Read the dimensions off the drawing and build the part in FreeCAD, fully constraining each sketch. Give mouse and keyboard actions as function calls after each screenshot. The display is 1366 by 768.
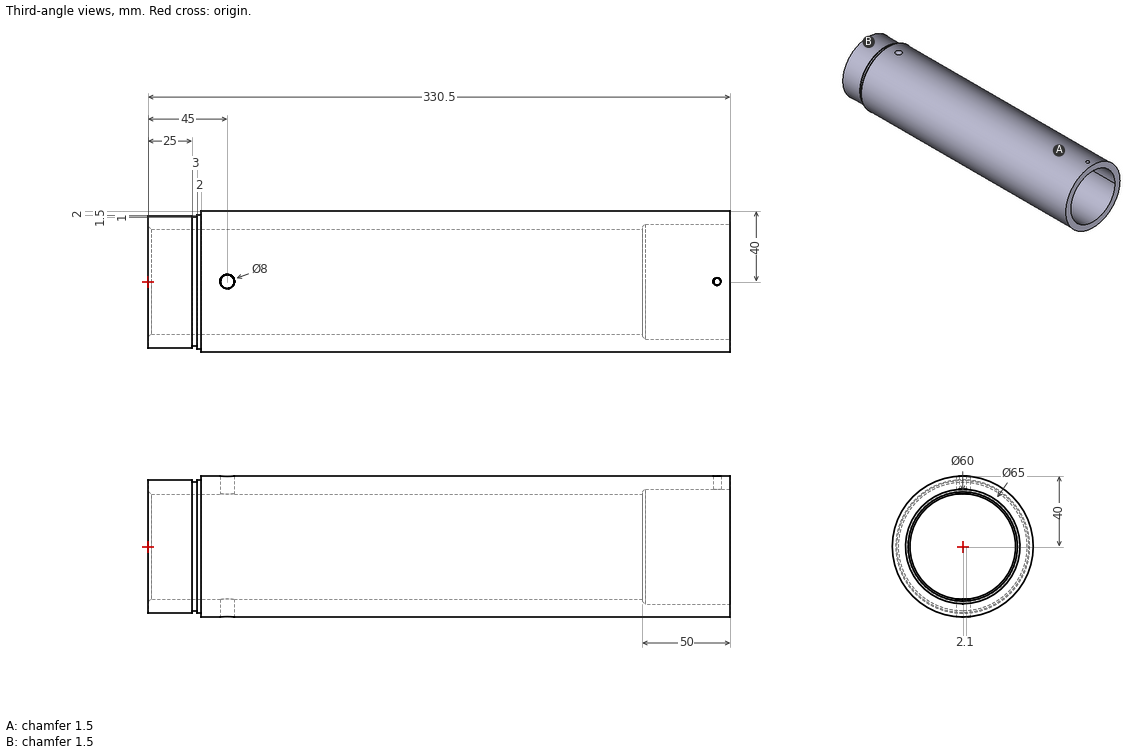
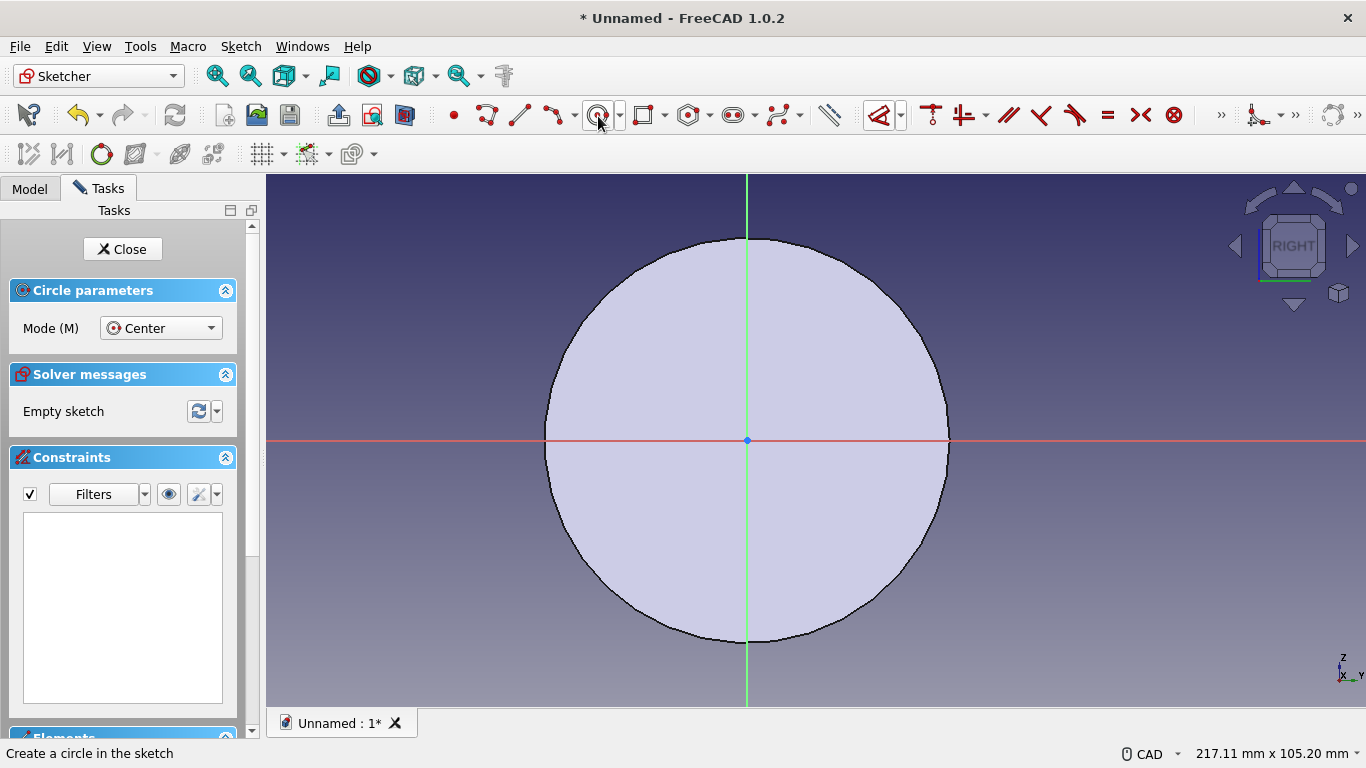
click(747, 440)
move(864, 324)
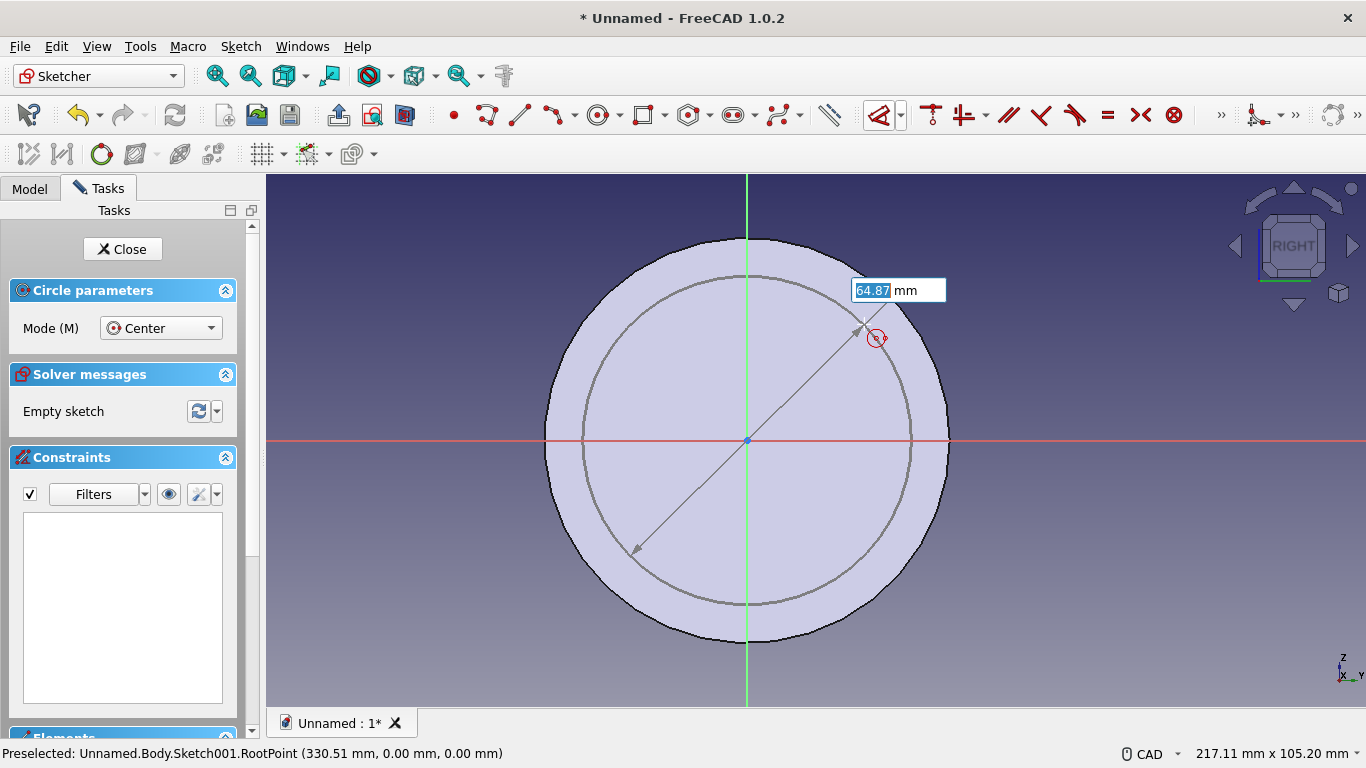
text(65)
key(Return)
key(Escape)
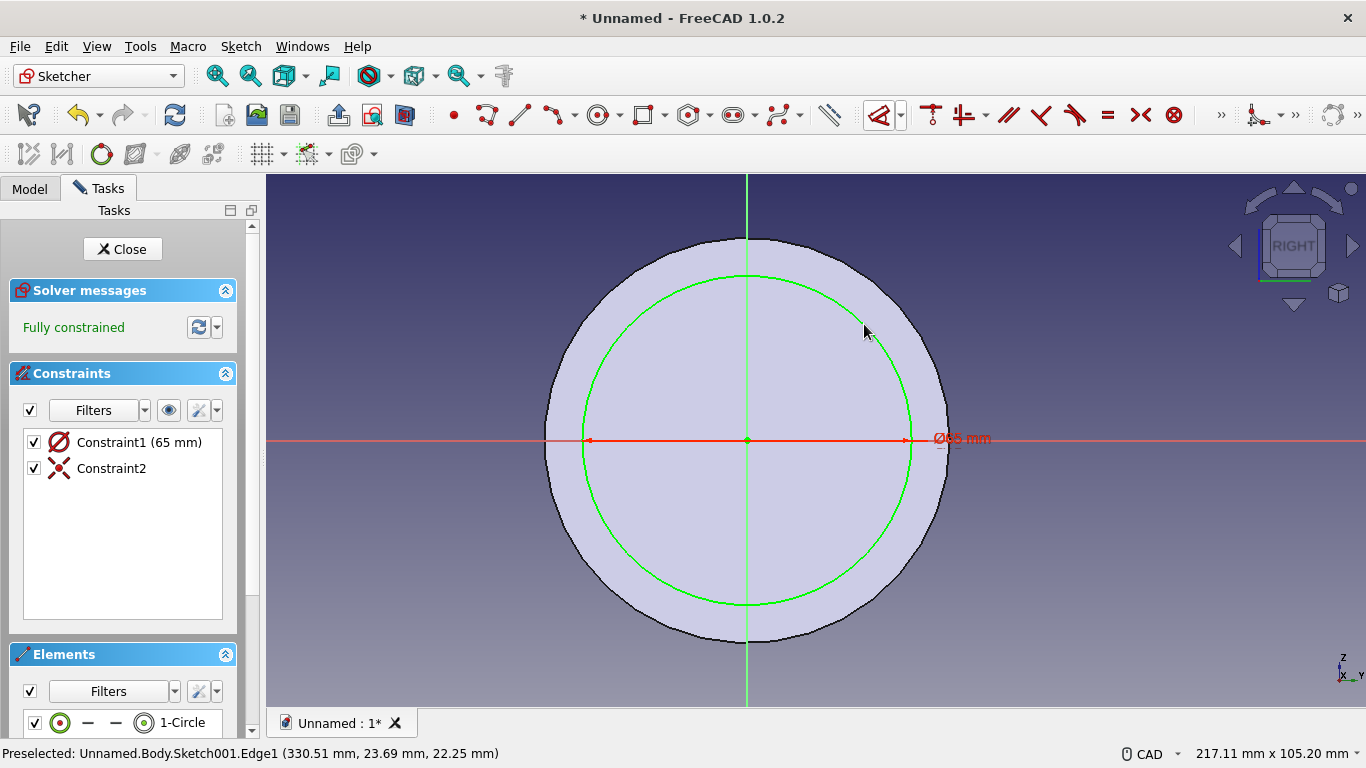
click(123, 249)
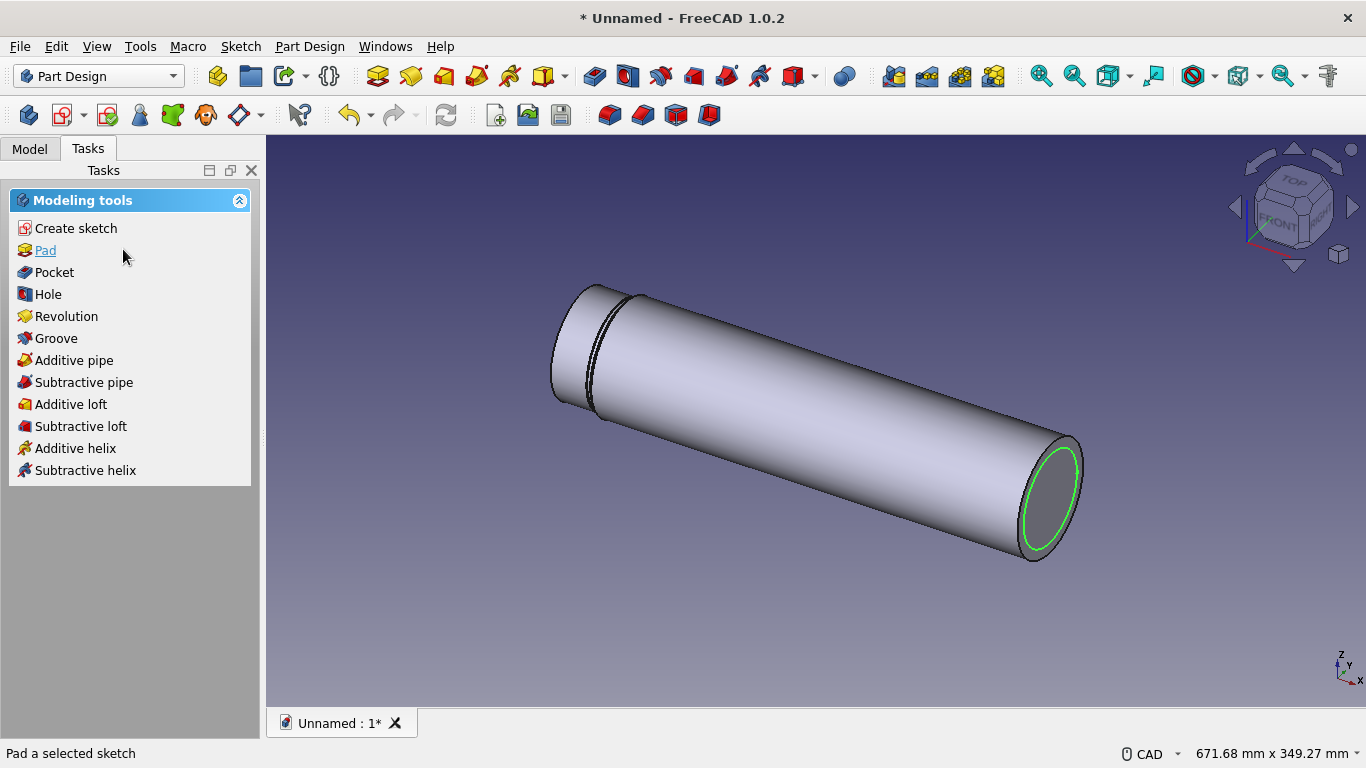
click(595, 76)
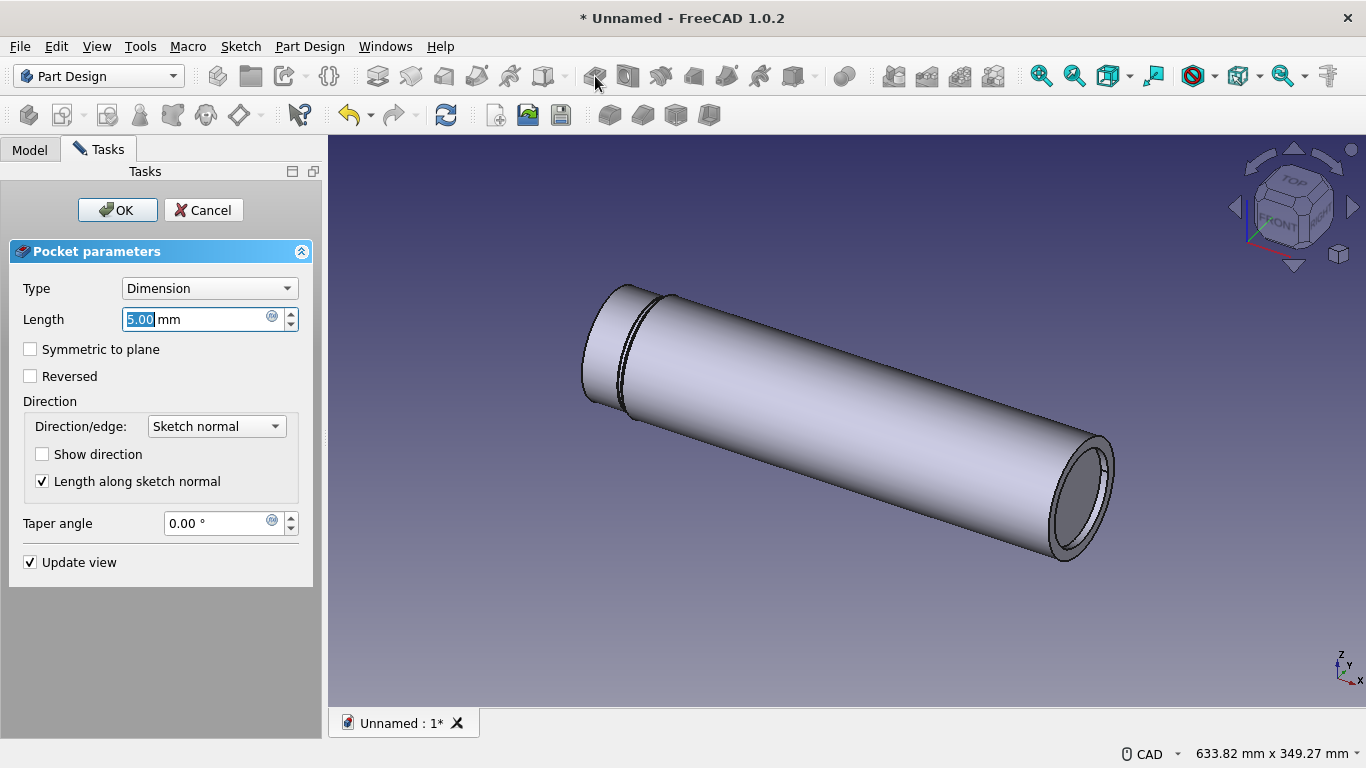
text(50)
key(Tab)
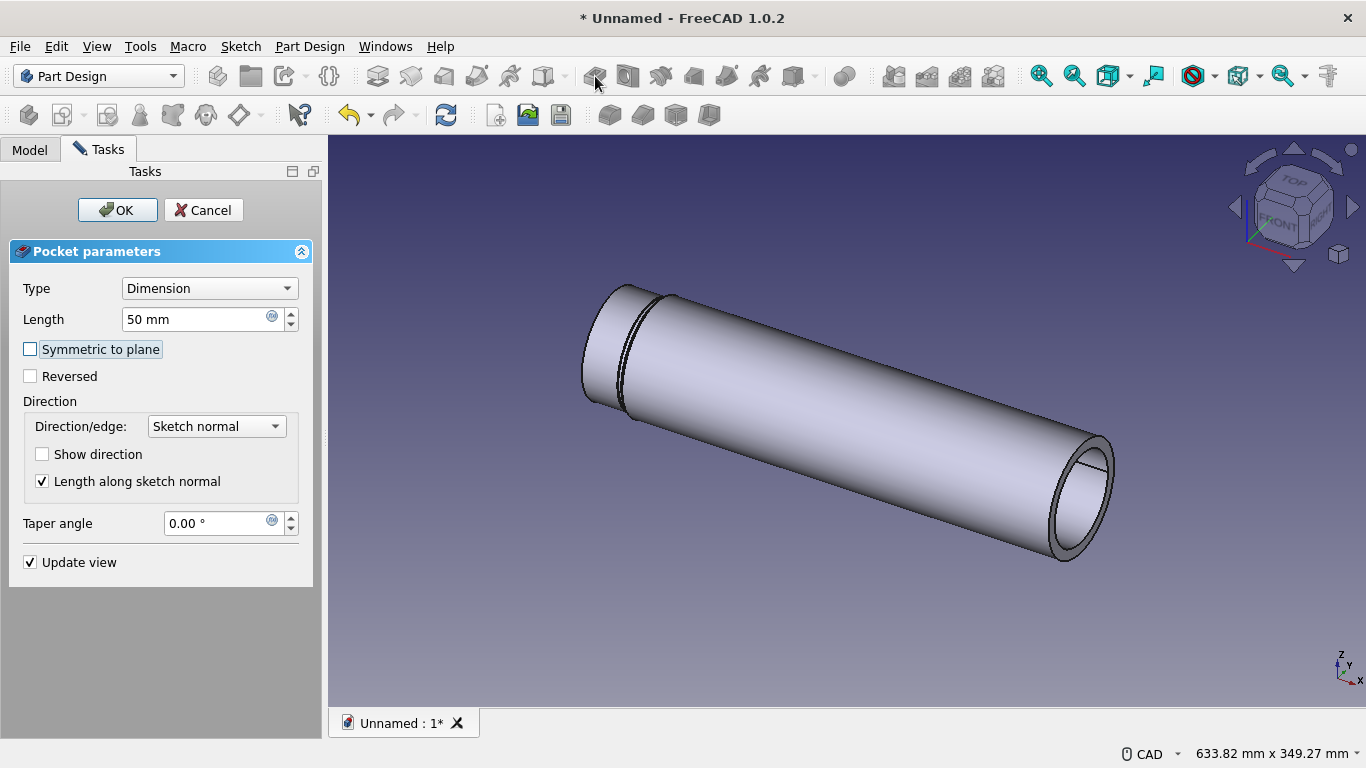
click(118, 210)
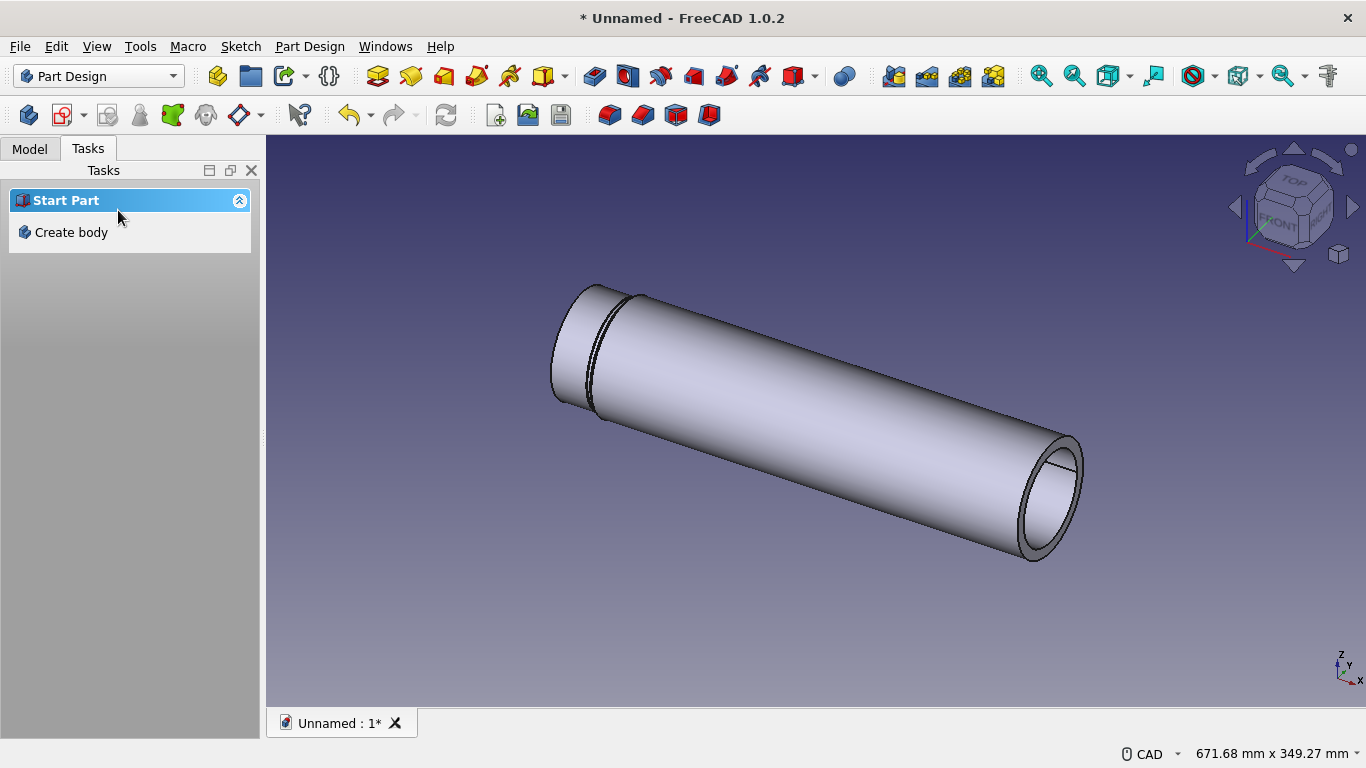
key(0)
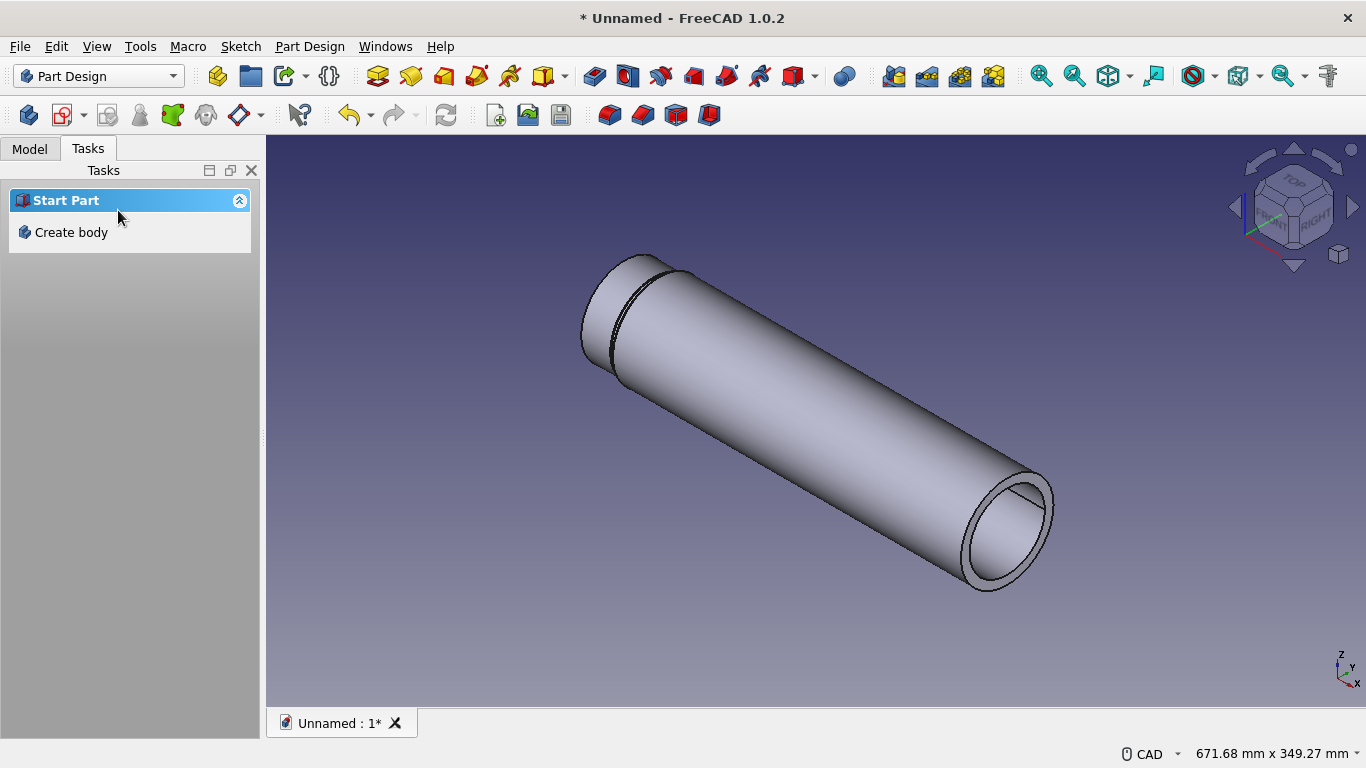
key(3)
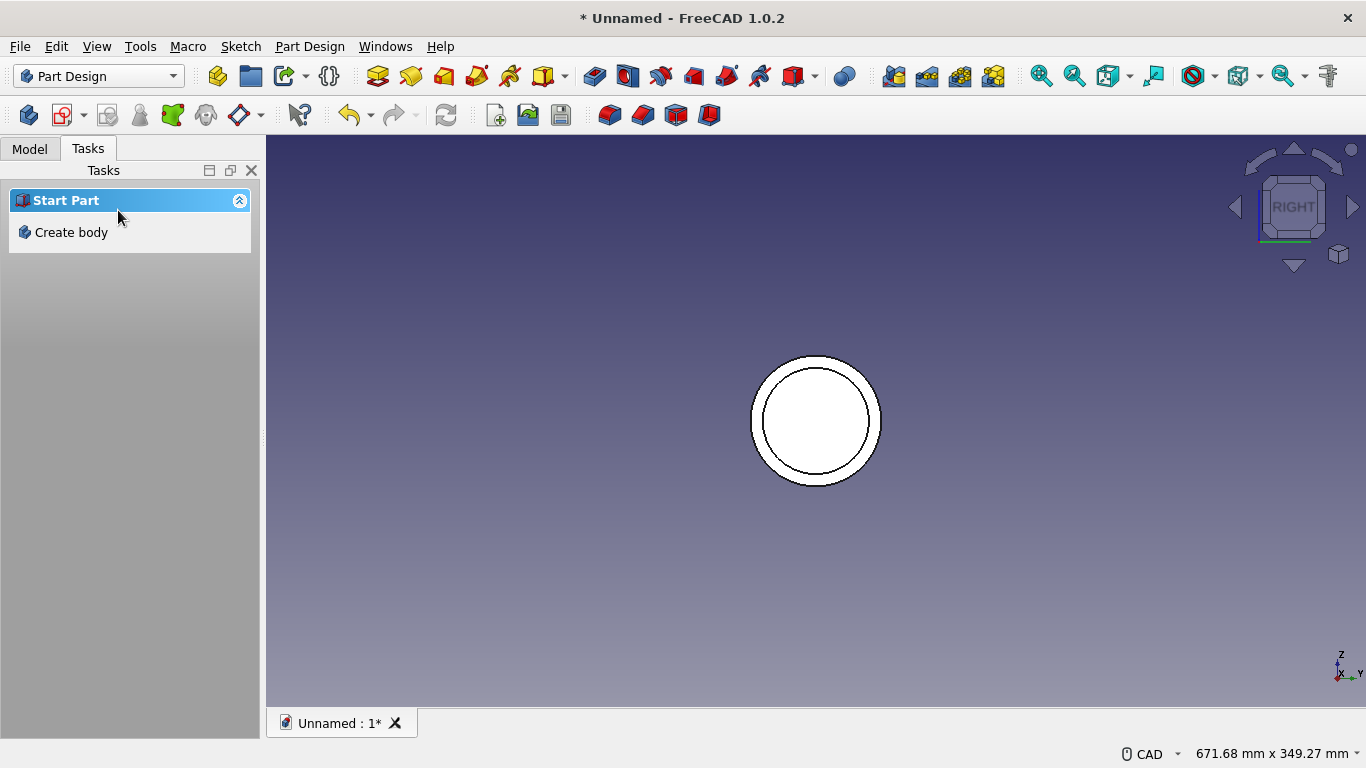
click(1042, 76)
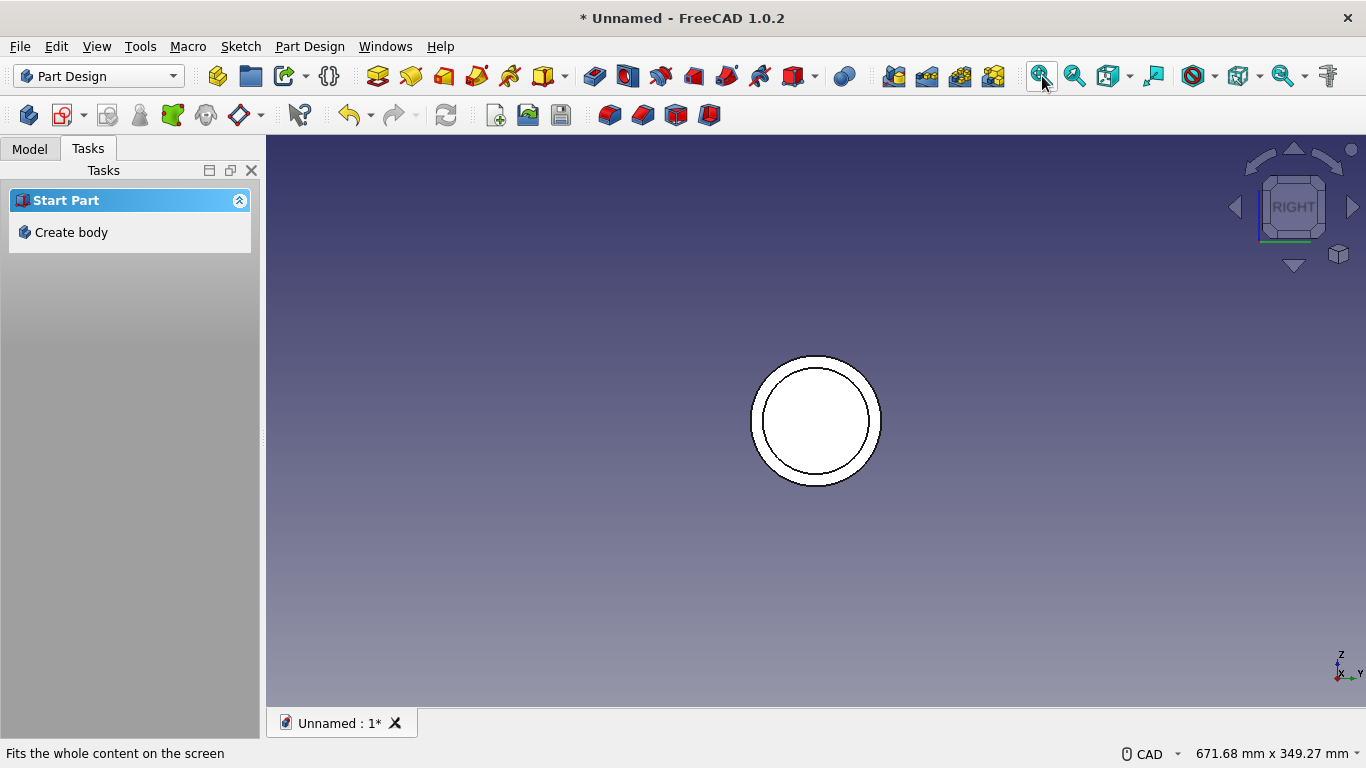
click(816, 420)